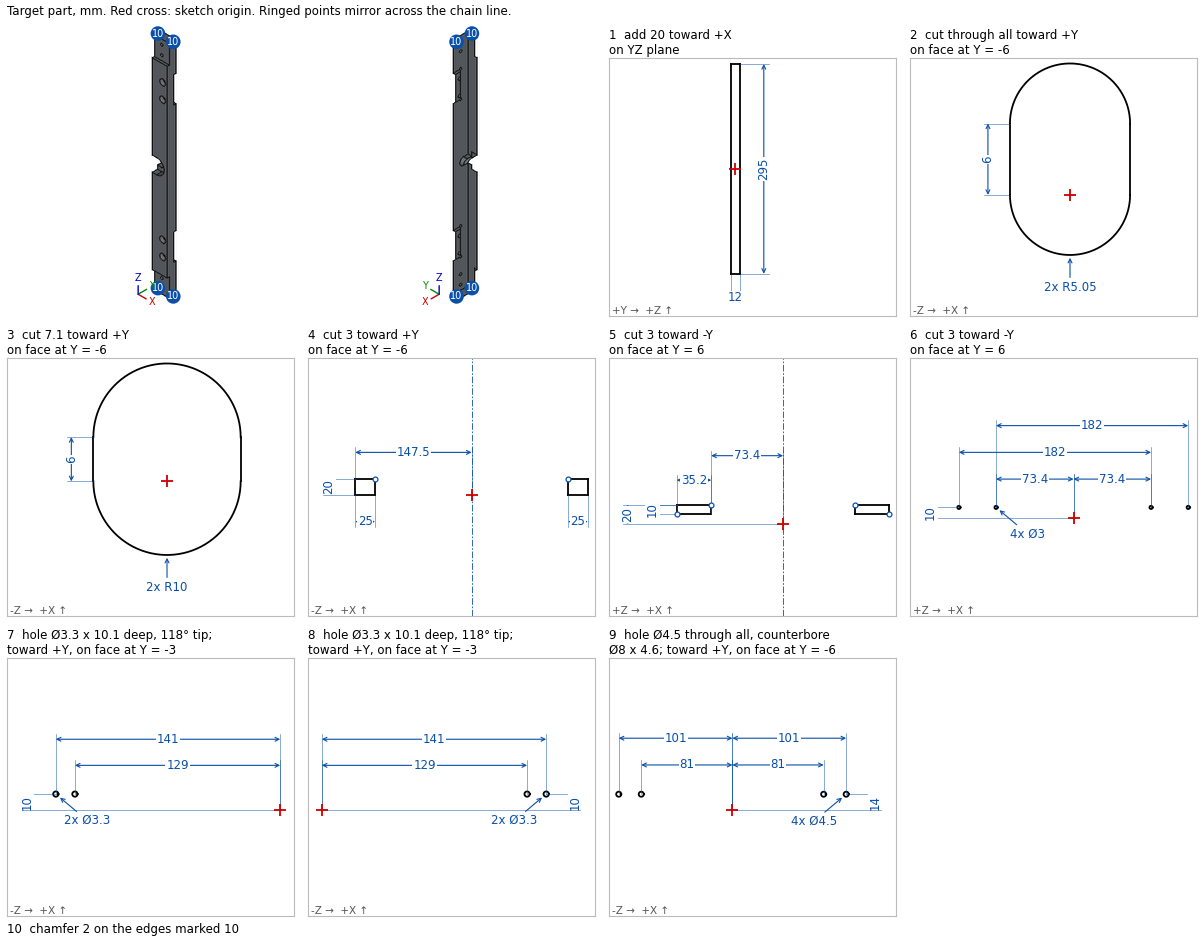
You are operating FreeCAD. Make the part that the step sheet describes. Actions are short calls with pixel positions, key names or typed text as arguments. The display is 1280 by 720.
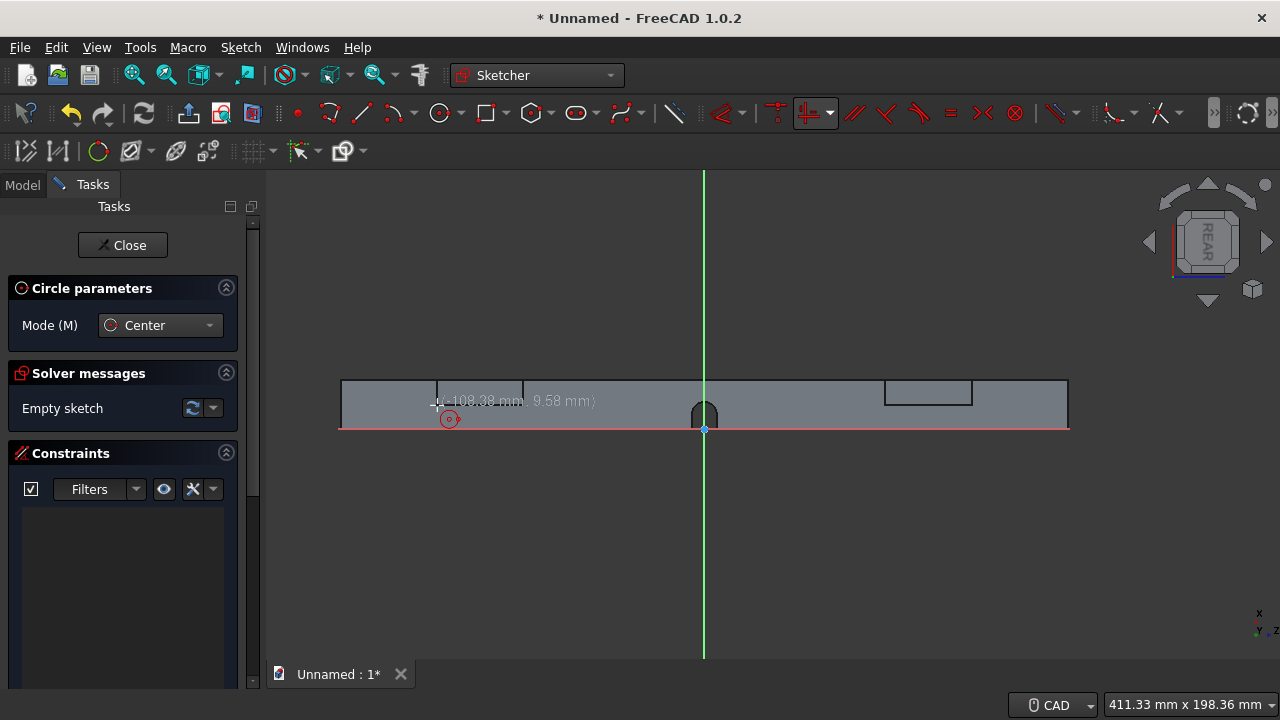
click(437, 405)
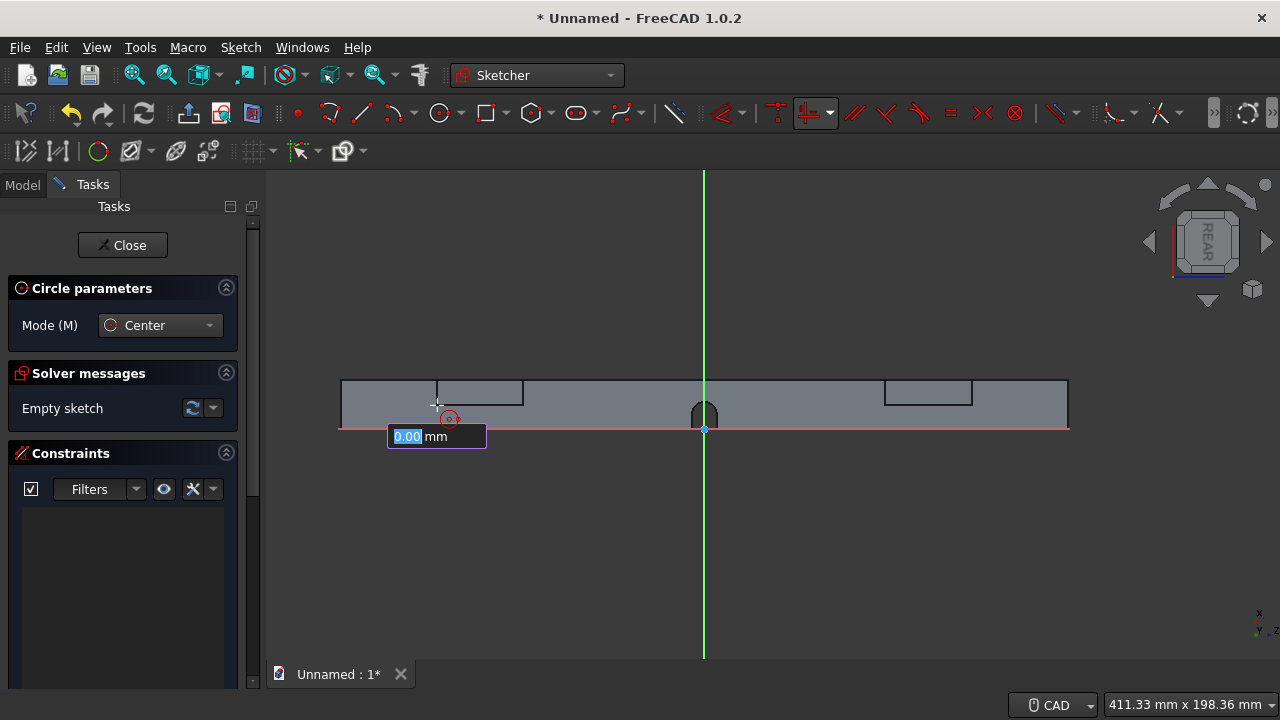
scroll(439, 402, up, 8)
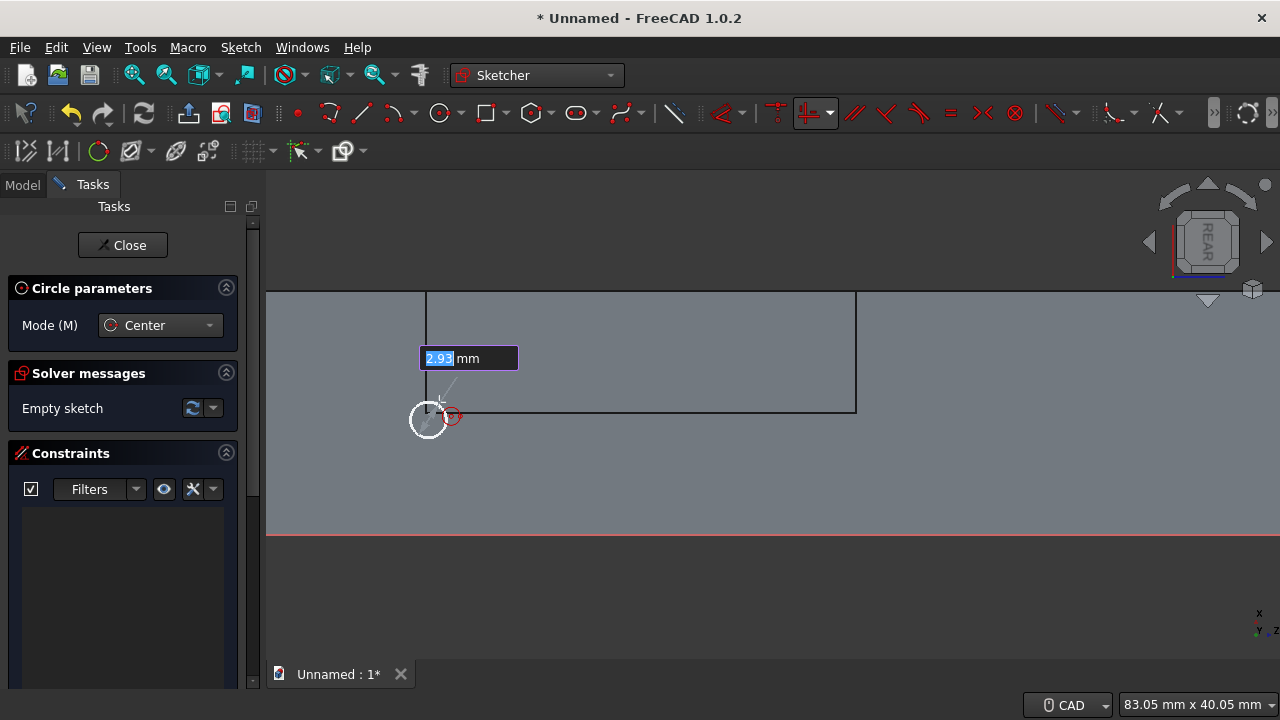
click(439, 400)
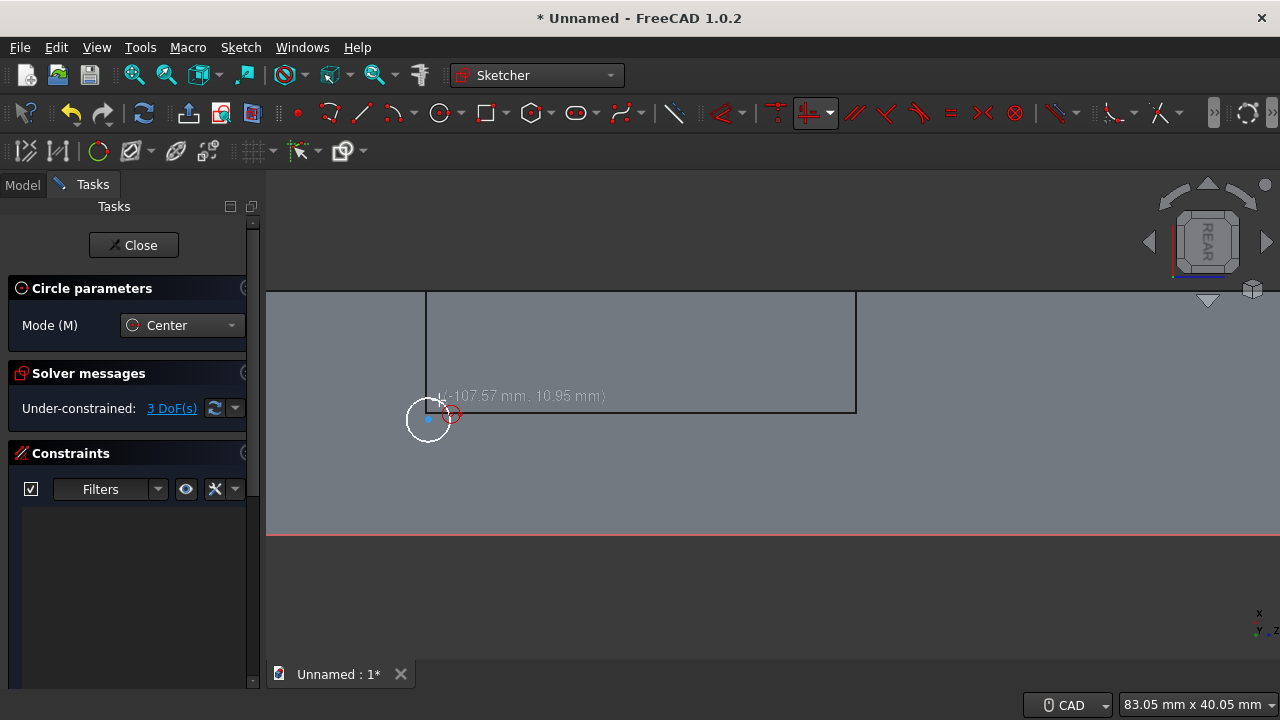
scroll(856, 413, up, 2)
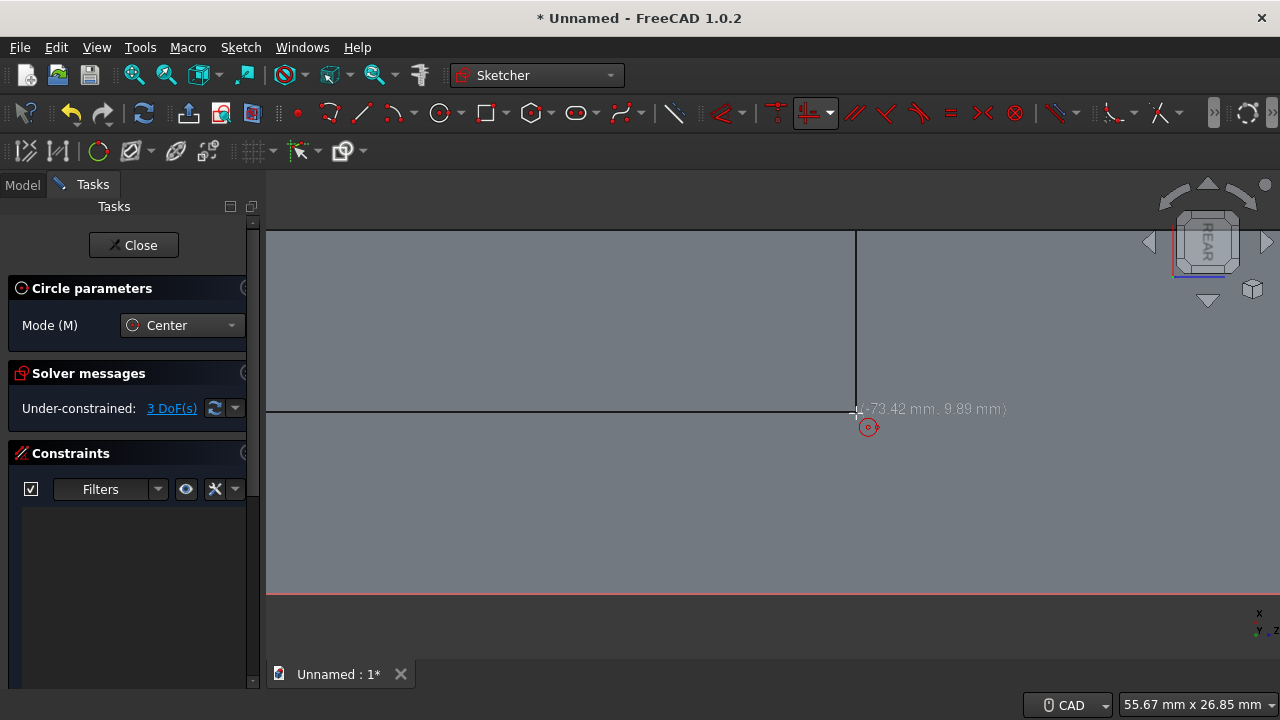
scroll(472, 403, down, 10)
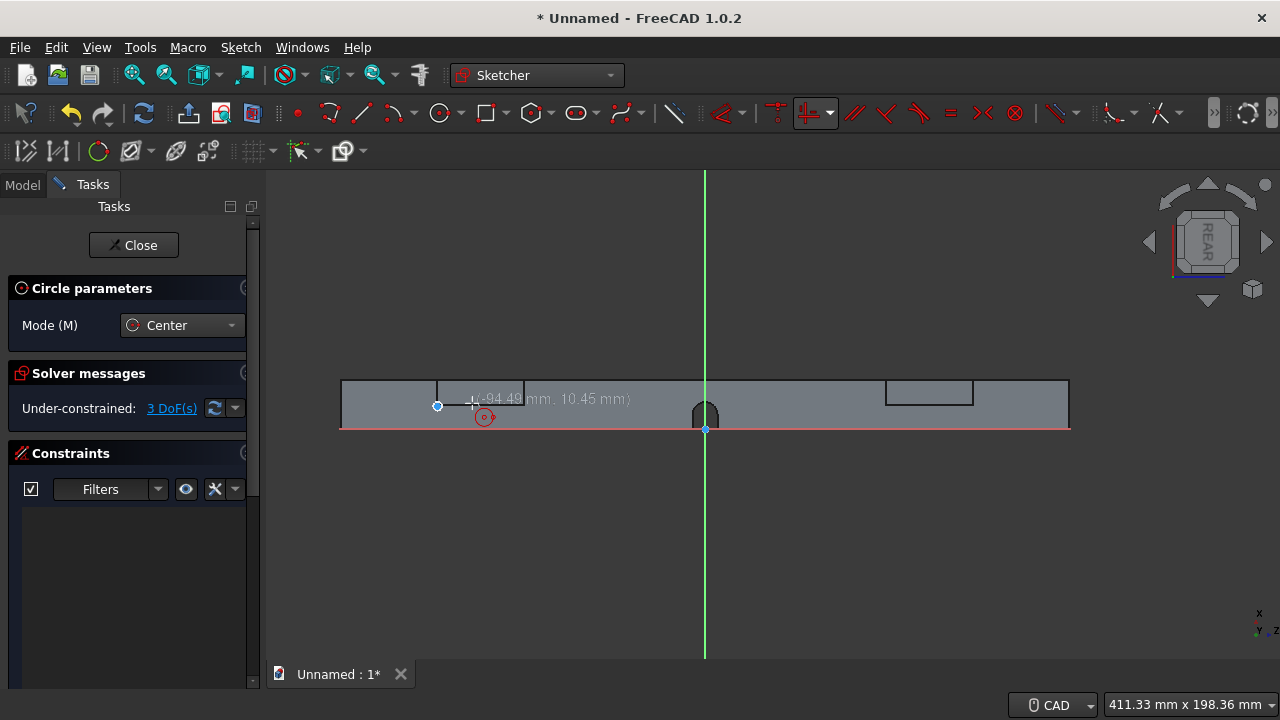
click(524, 405)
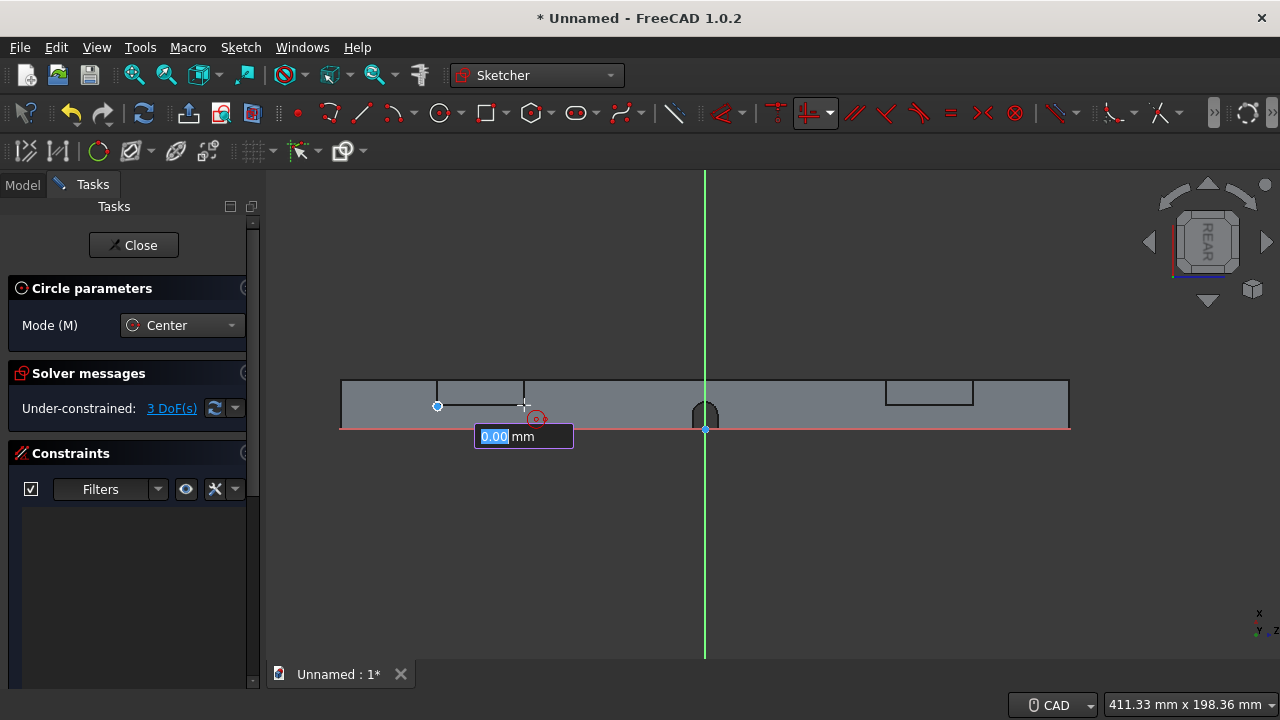
scroll(527, 402, up, 8)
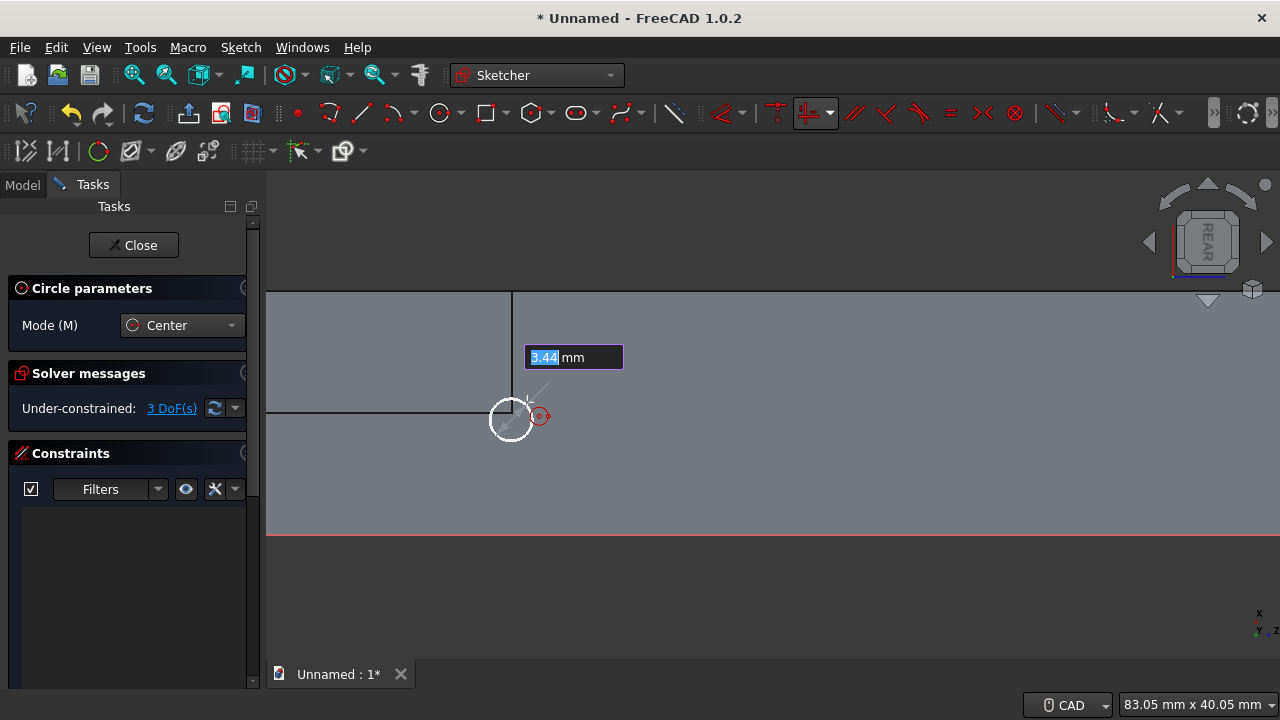
click(525, 400)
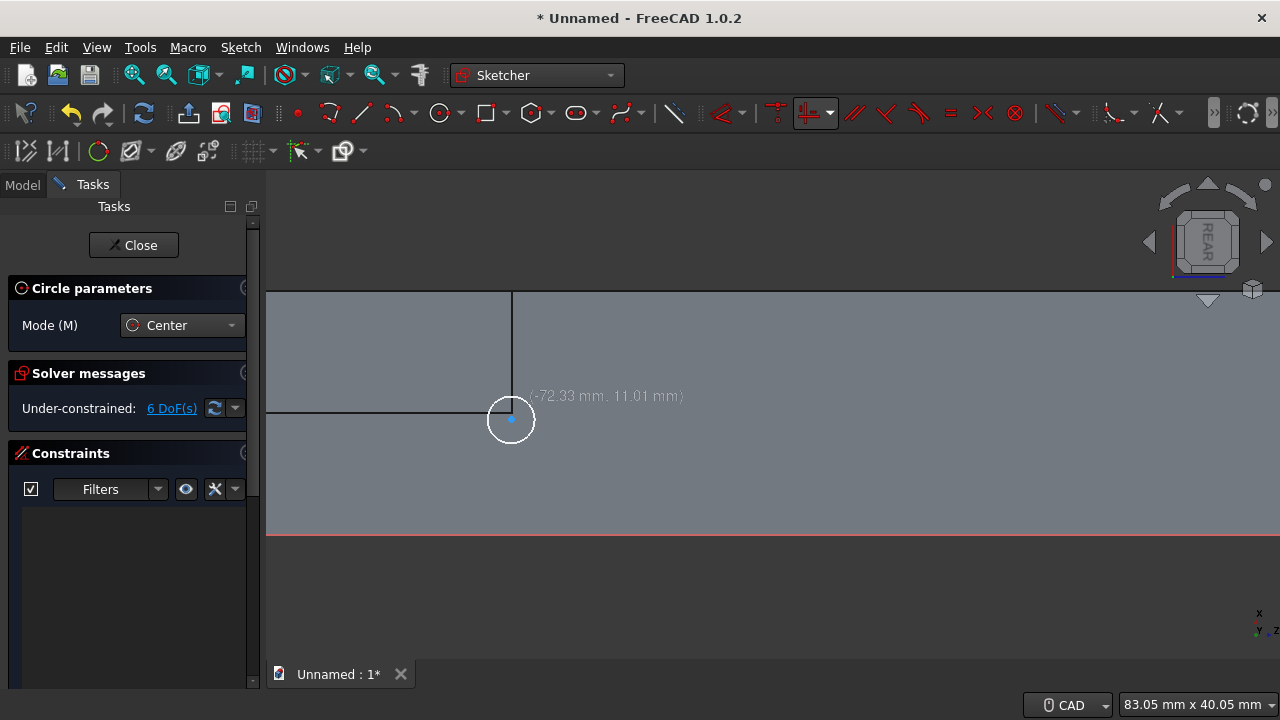
scroll(527, 402, down, 8)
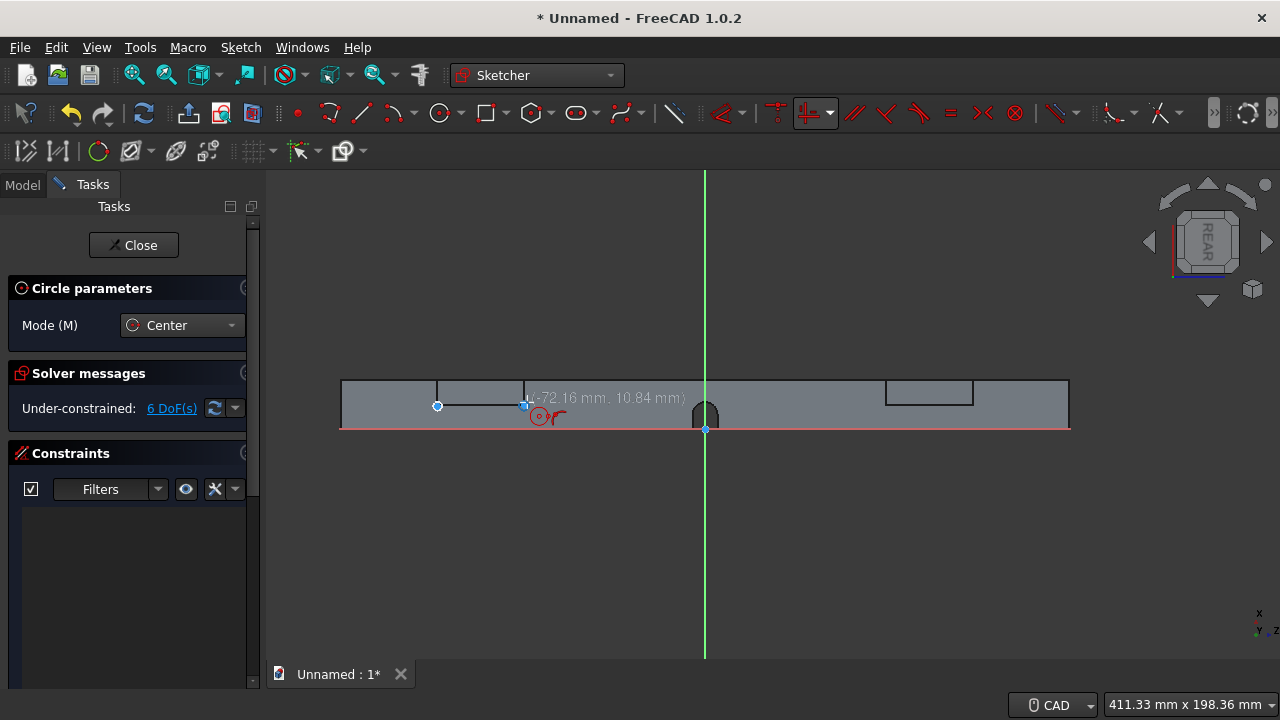
scroll(886, 405, up, 10)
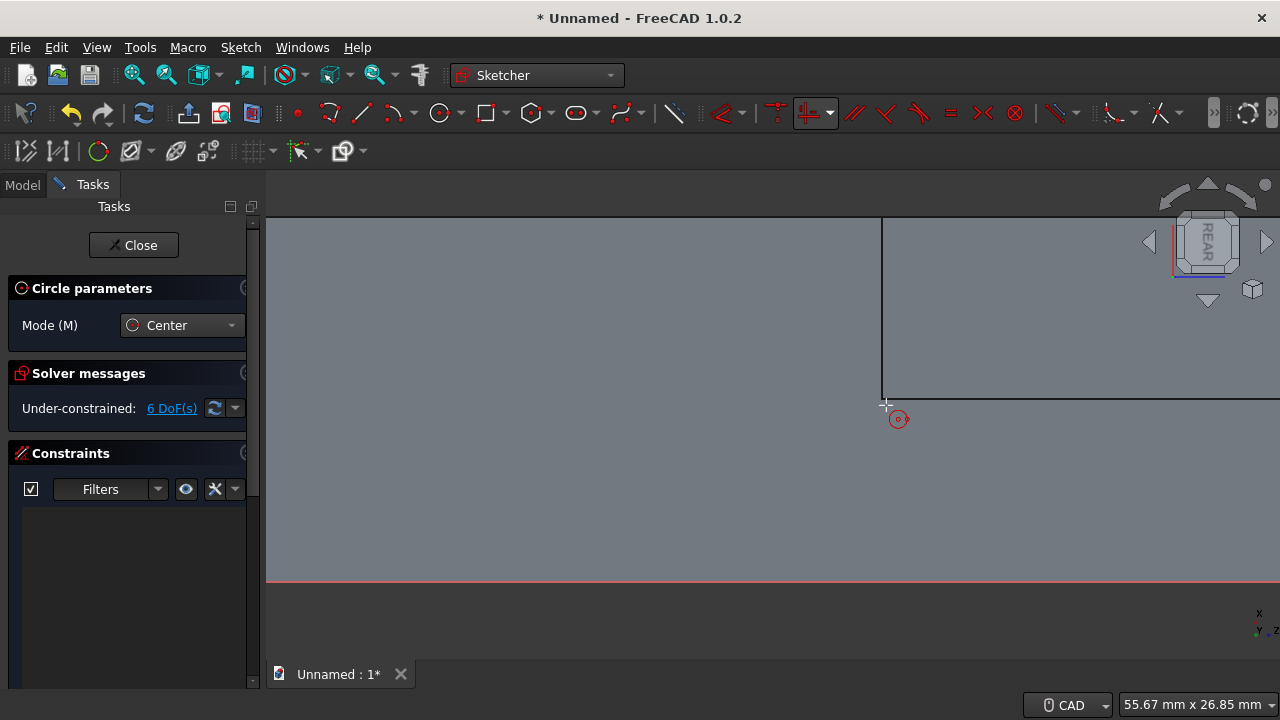
scroll(886, 405, down, 10)